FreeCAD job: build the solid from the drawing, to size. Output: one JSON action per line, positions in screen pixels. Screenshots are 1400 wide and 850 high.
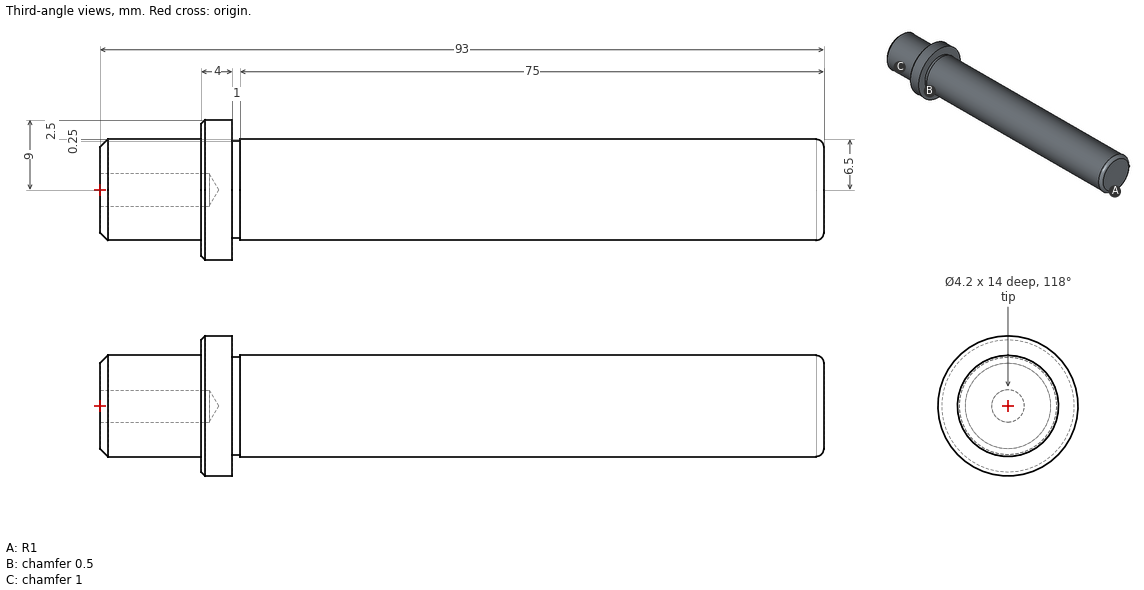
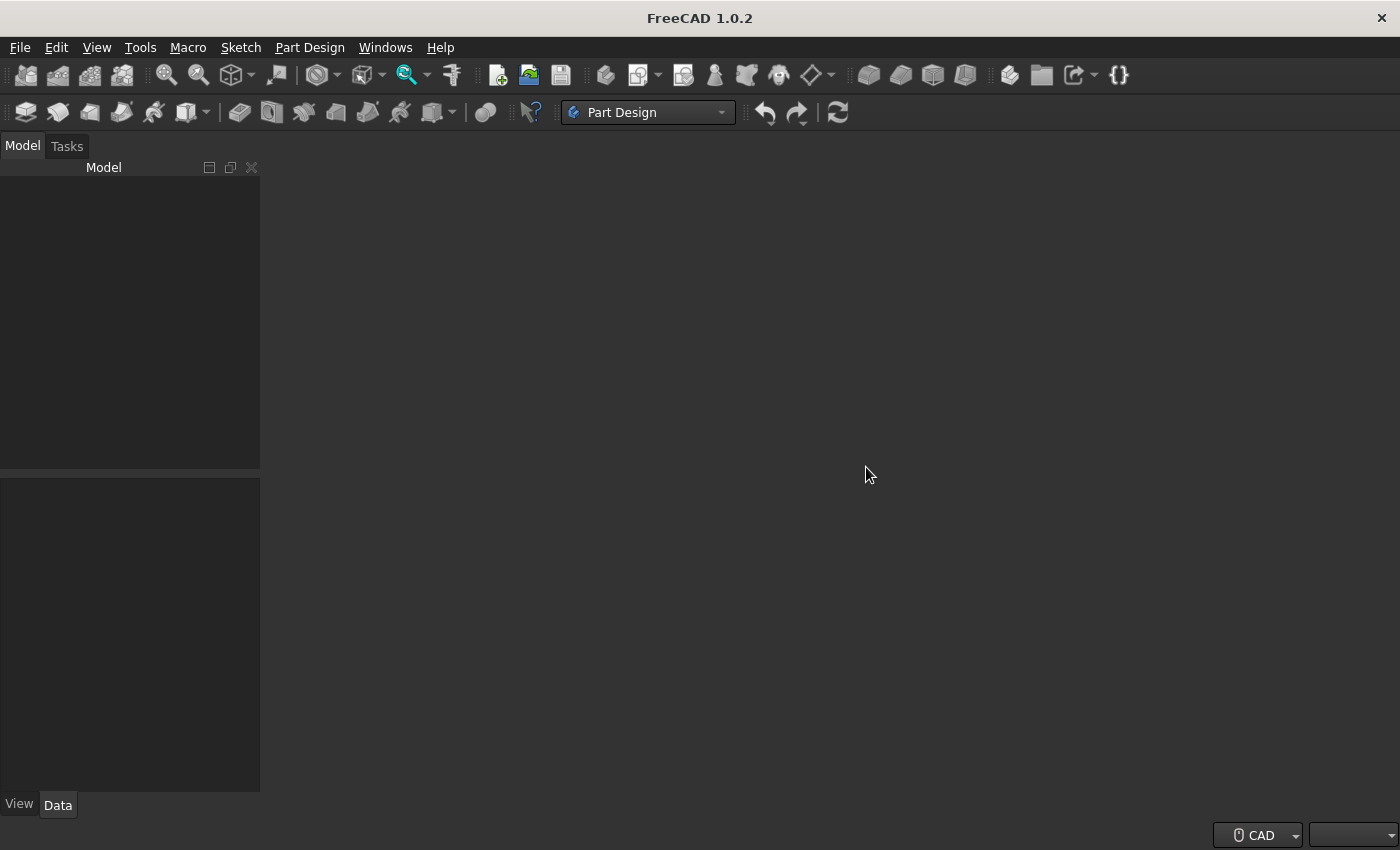
{"action": "key", "text": "ctrl+n"}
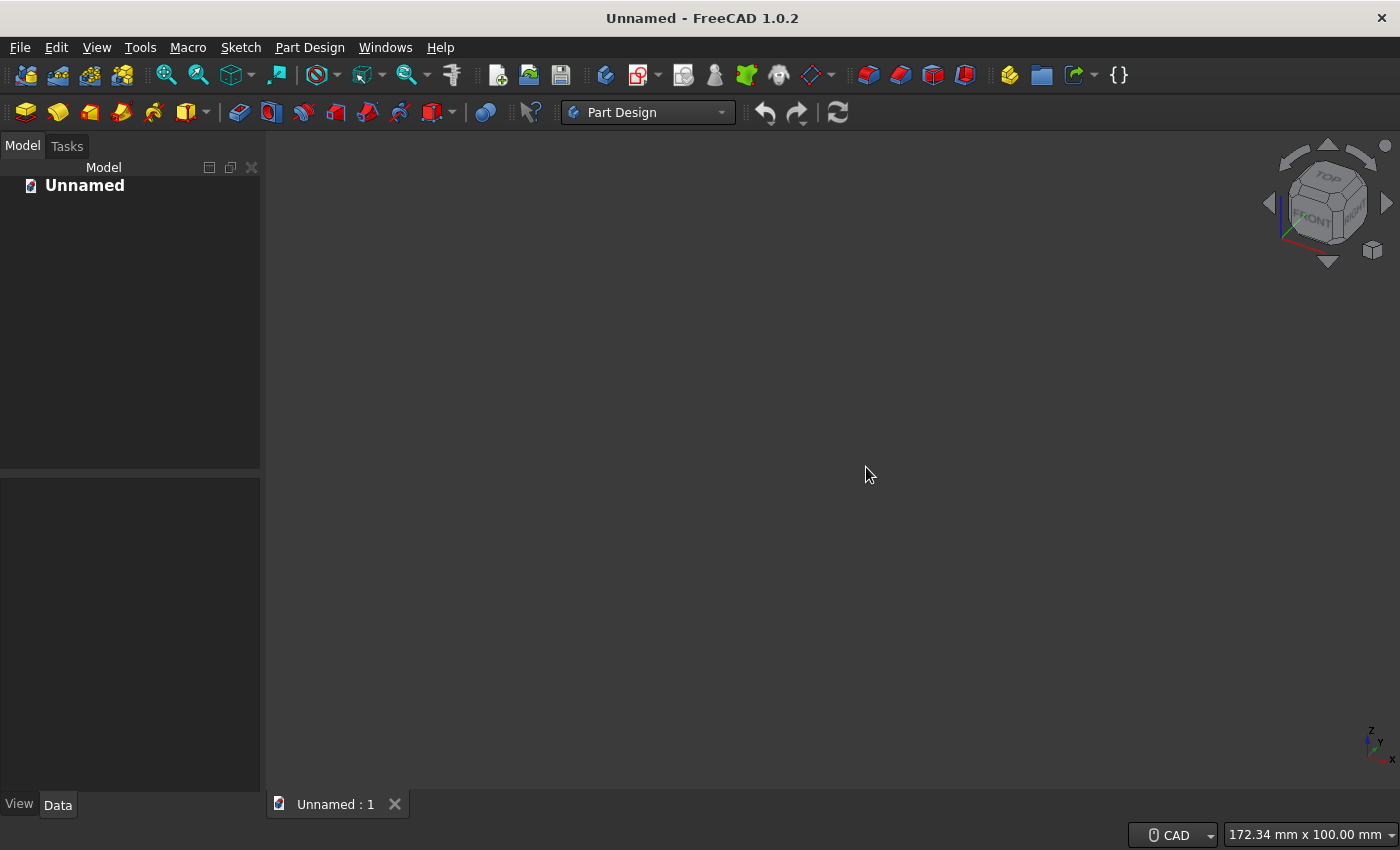
{"action": "left_click", "coordinate": [638, 76]}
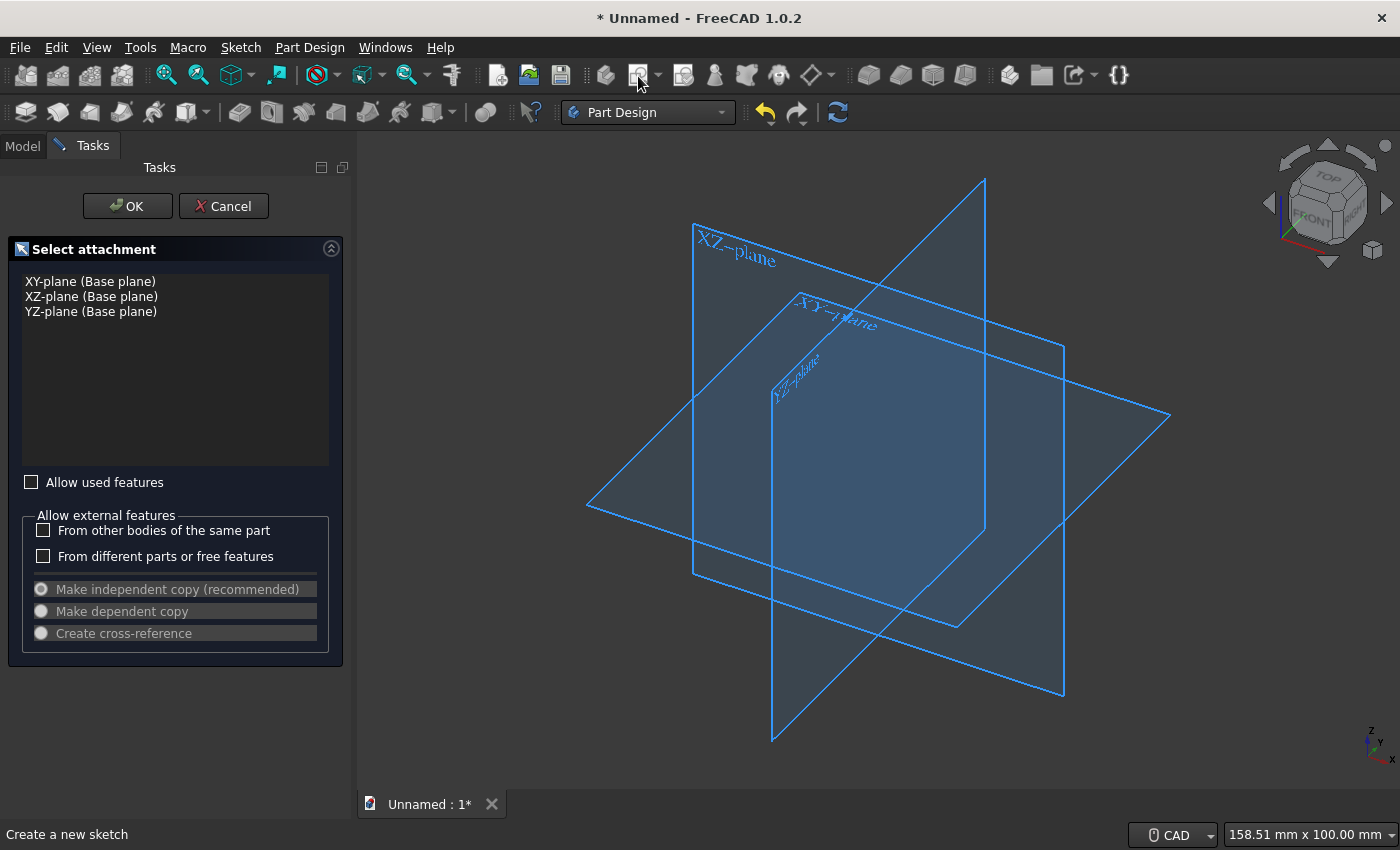
{"action": "left_click", "coordinate": [82, 282]}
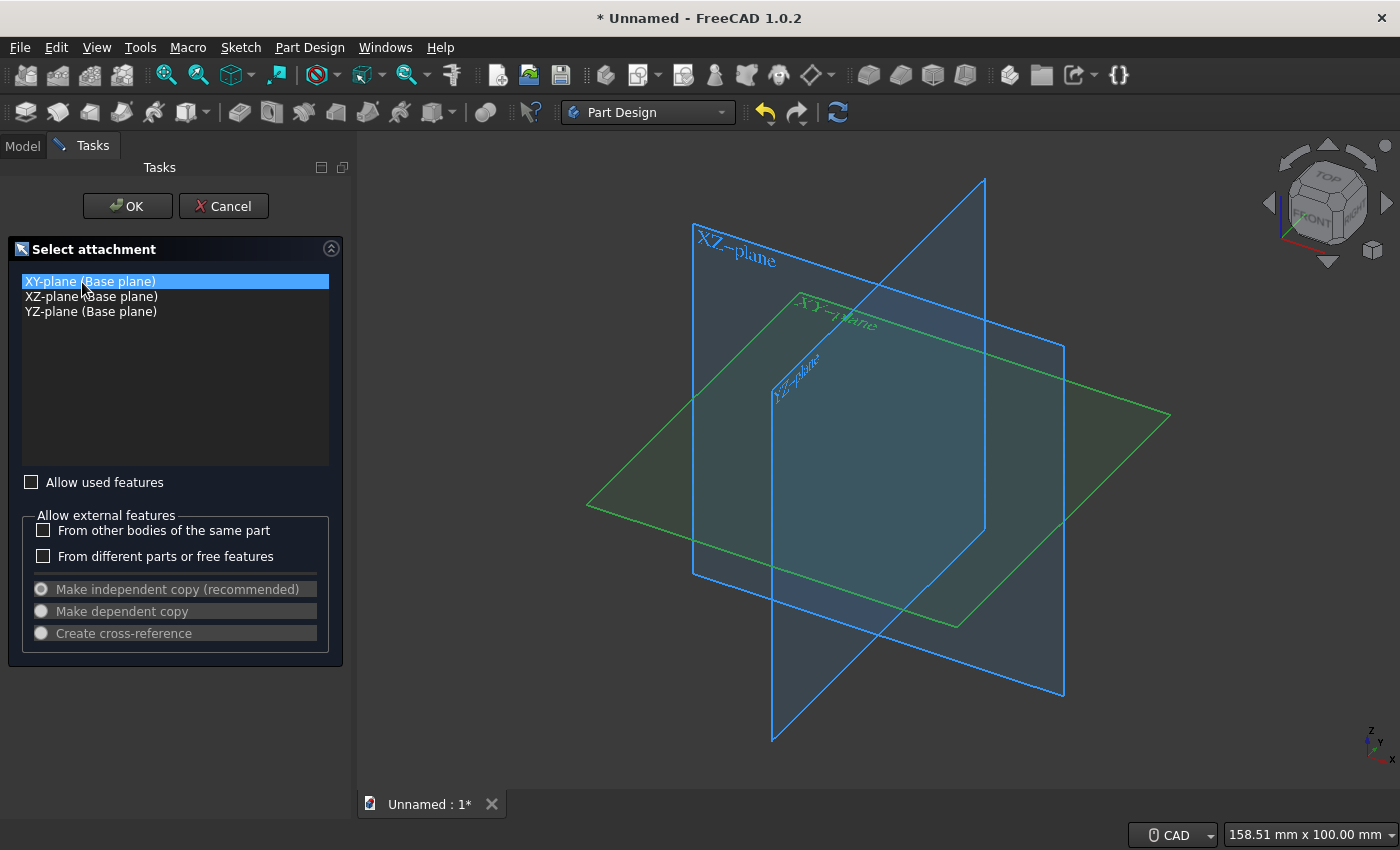
{"action": "left_click", "coordinate": [128, 206]}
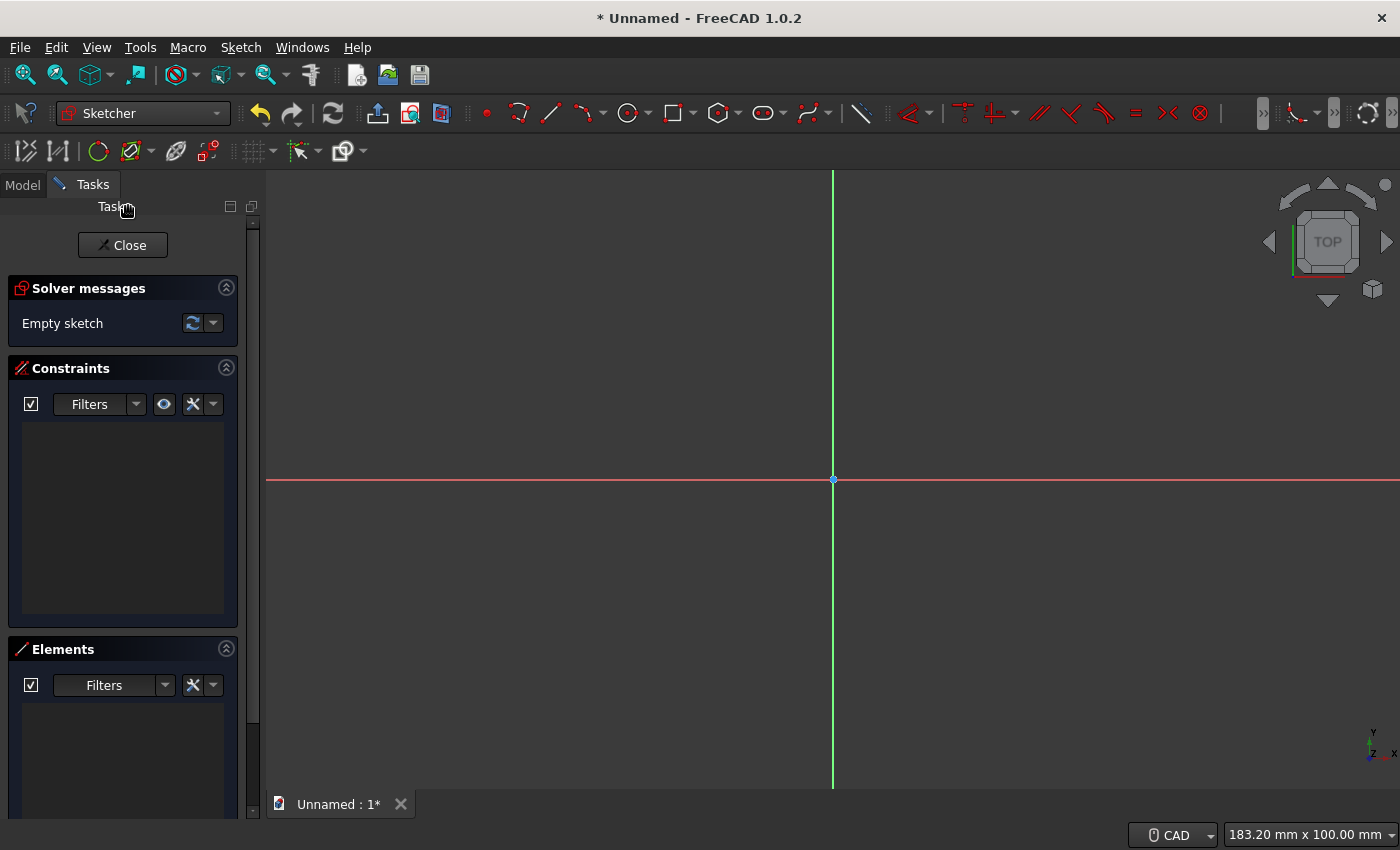
{"action": "scroll", "coordinate": [294, 605], "scroll_direction": "down", "scroll_amount": 1}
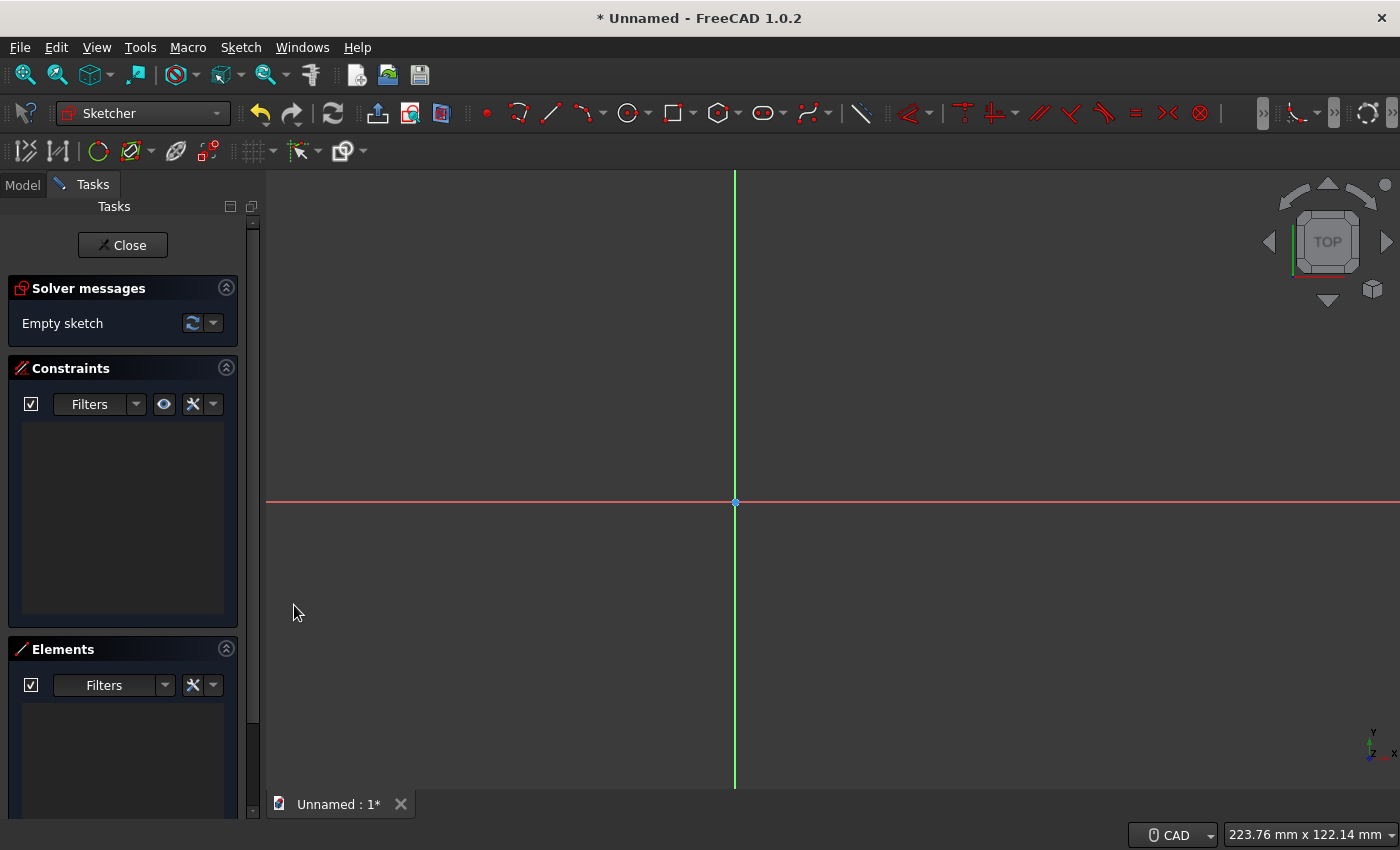
{"action": "scroll", "coordinate": [1235, 480], "scroll_direction": "up", "scroll_amount": 2}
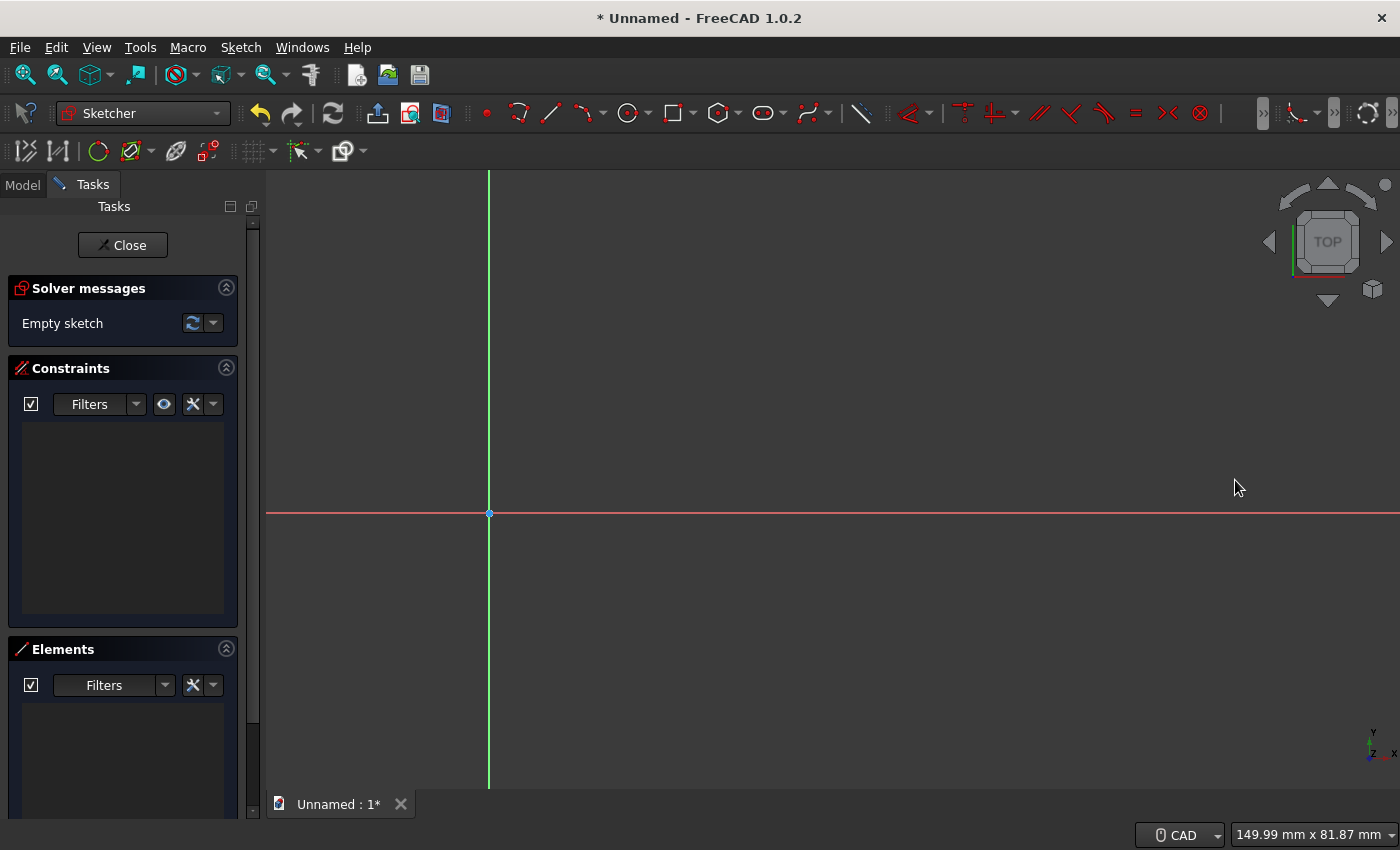
{"action": "left_click", "coordinate": [520, 114]}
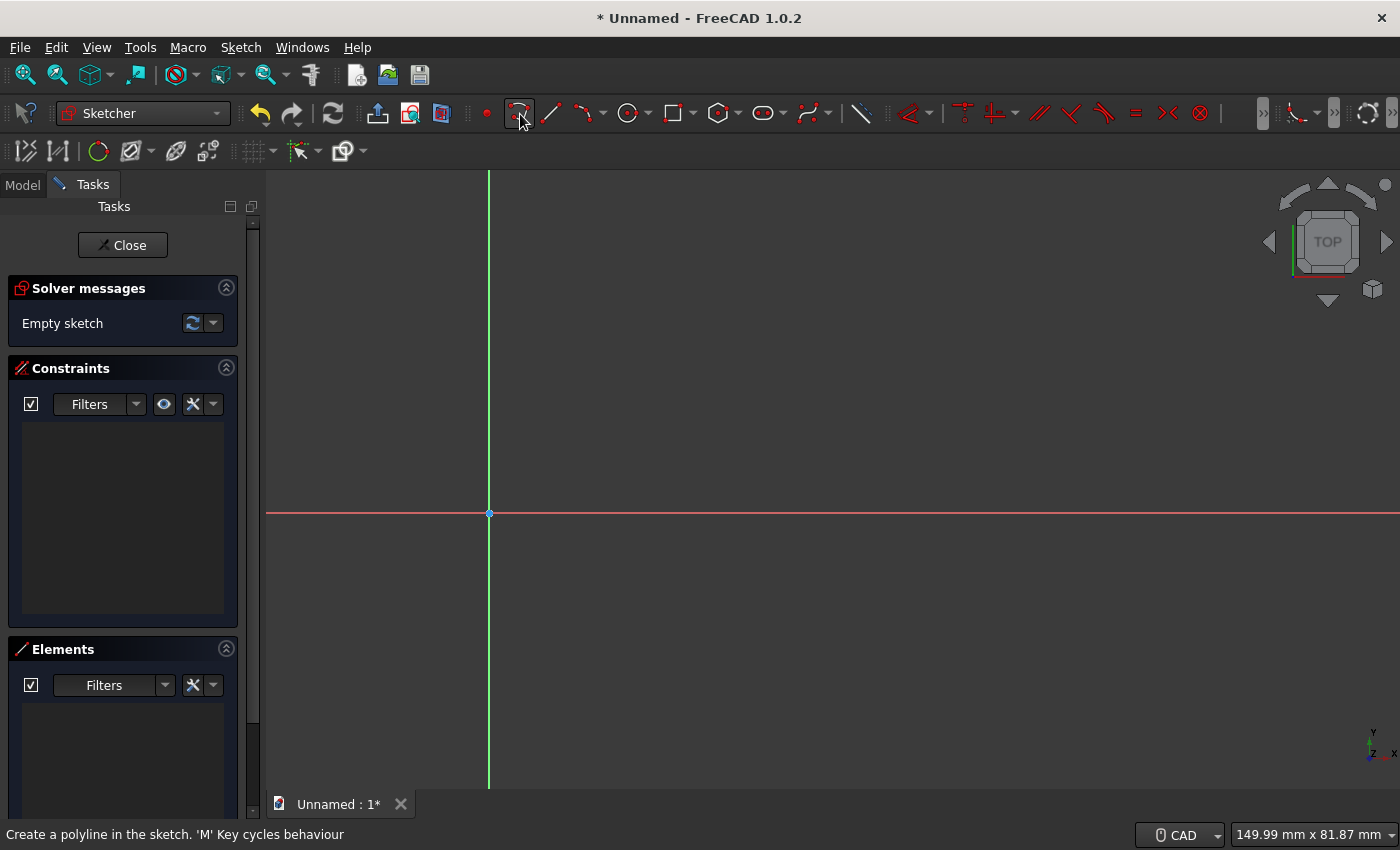
{"action": "left_click", "coordinate": [489, 513]}
{"action": "left_click", "coordinate": [1192, 504]}
{"action": "left_click", "coordinate": [1192, 464]}
{"action": "left_click", "coordinate": [625, 464]}